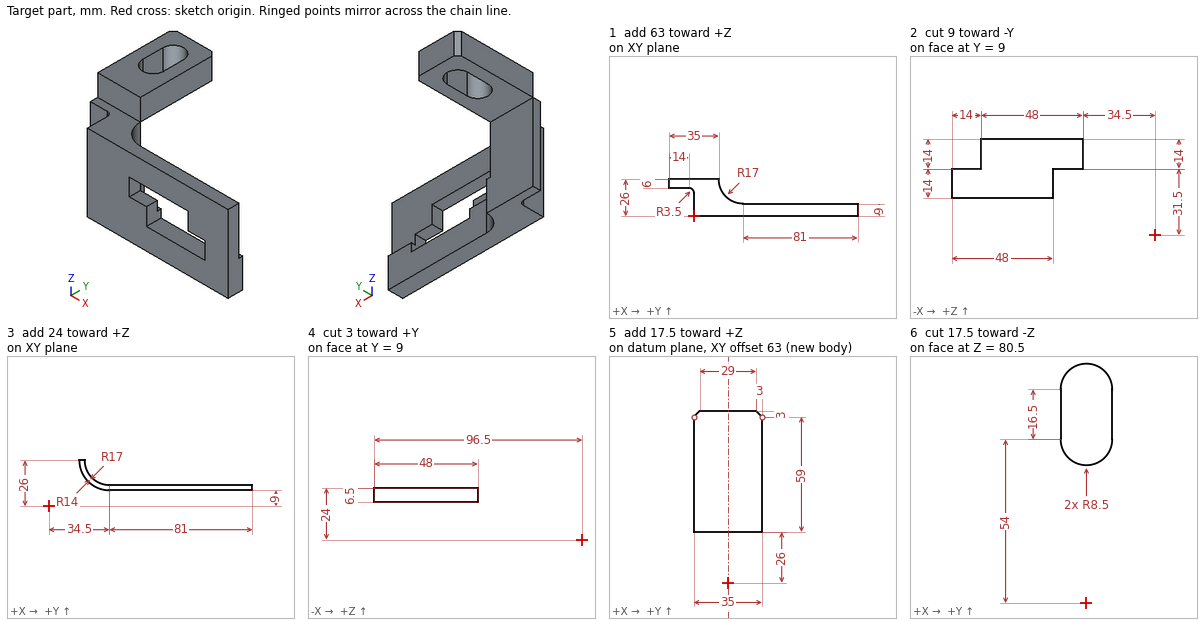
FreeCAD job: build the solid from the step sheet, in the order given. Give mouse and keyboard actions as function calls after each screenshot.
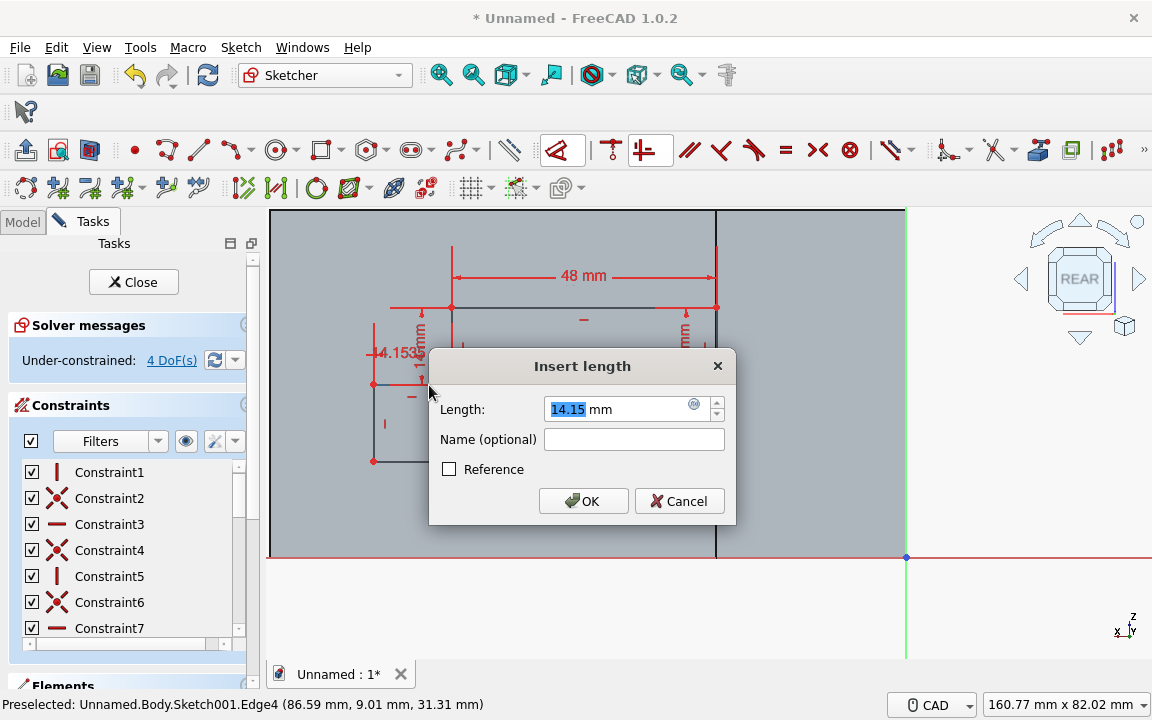
text(14)
key(Return)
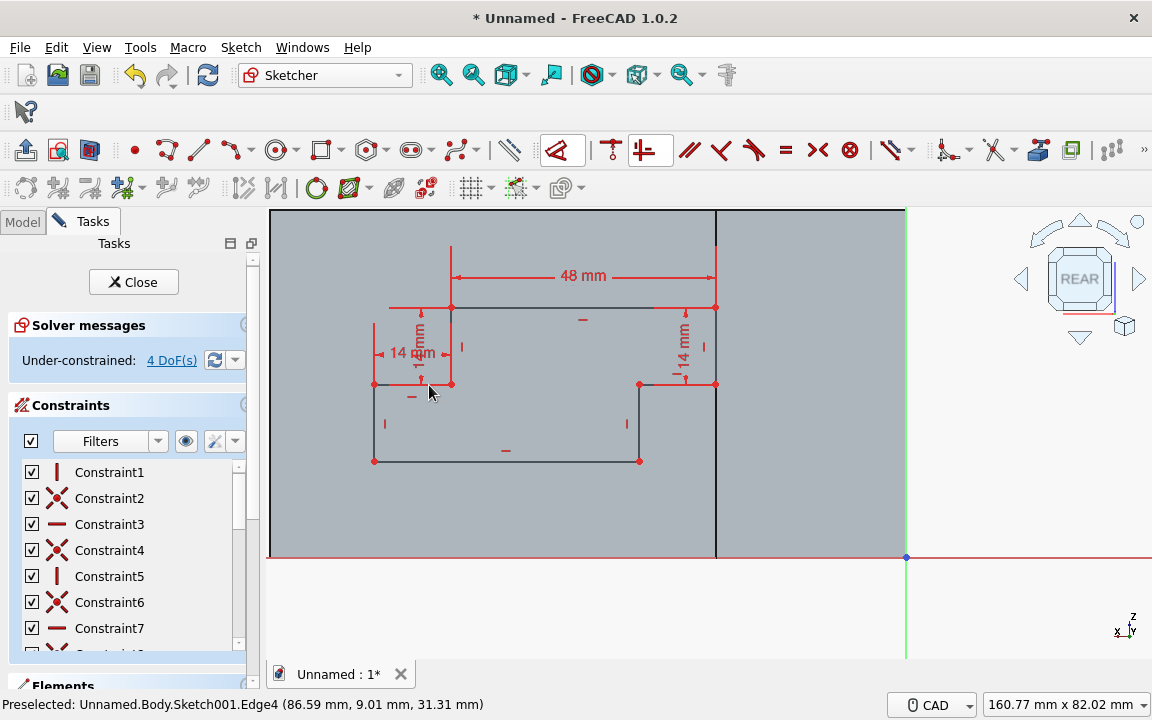
click(374, 408)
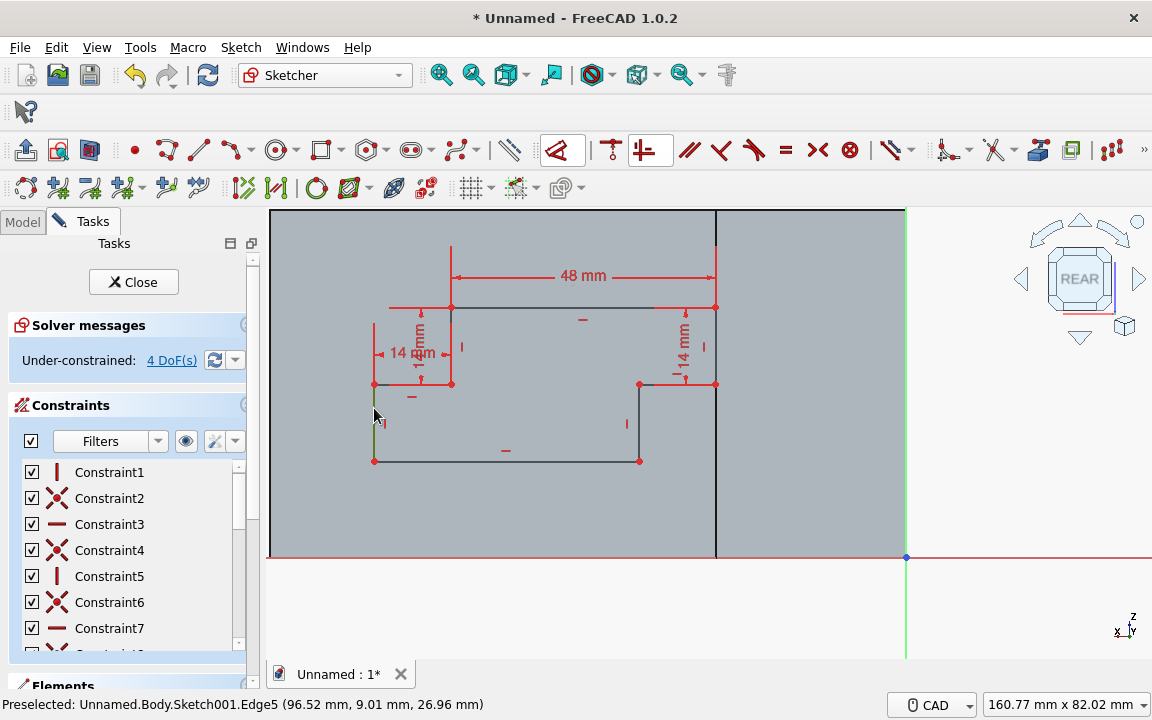
key(i)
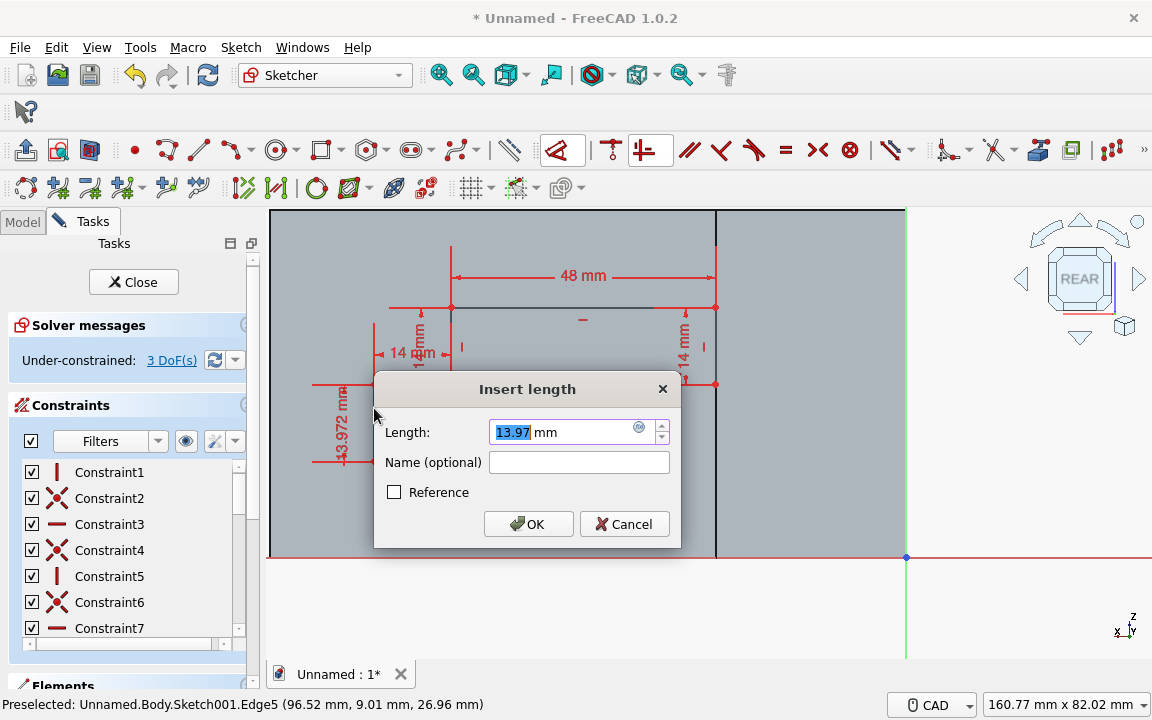
text(14)
key(Return)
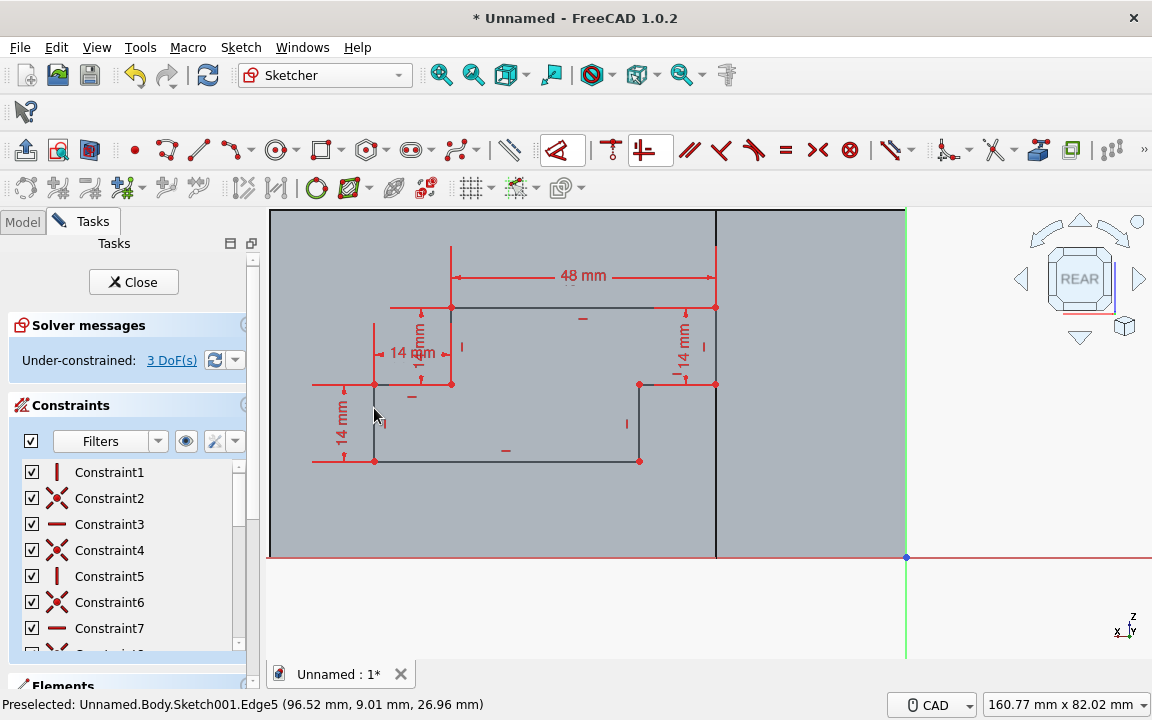
click(454, 462)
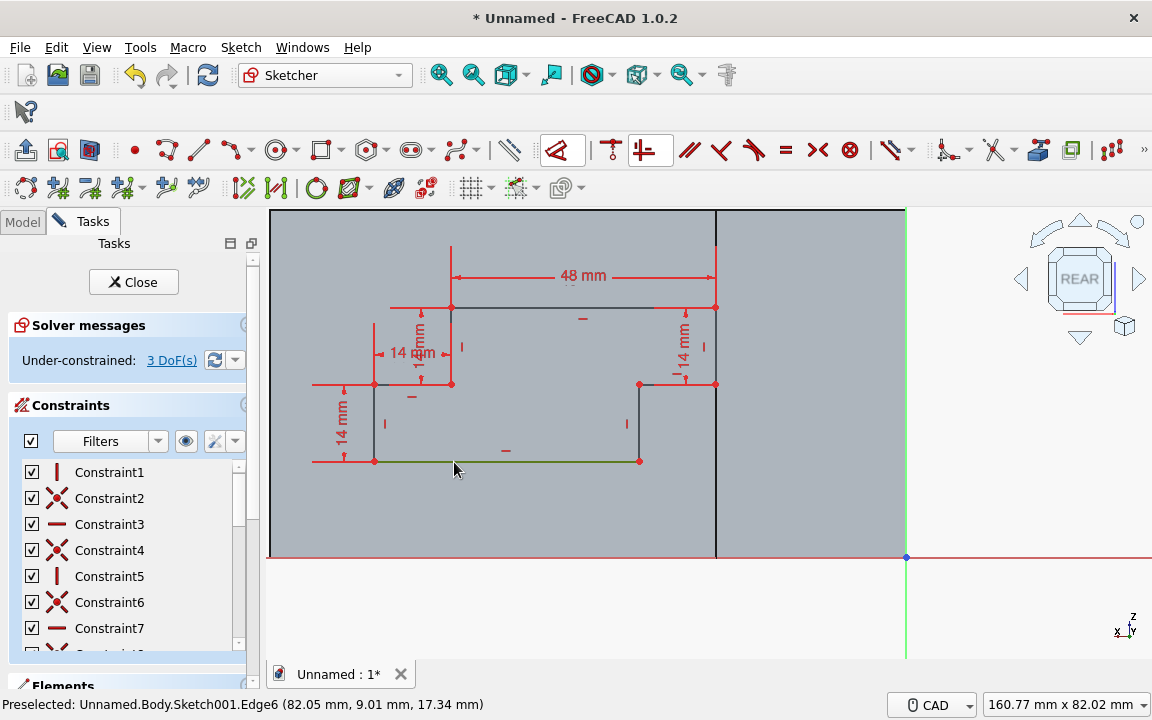
key(l)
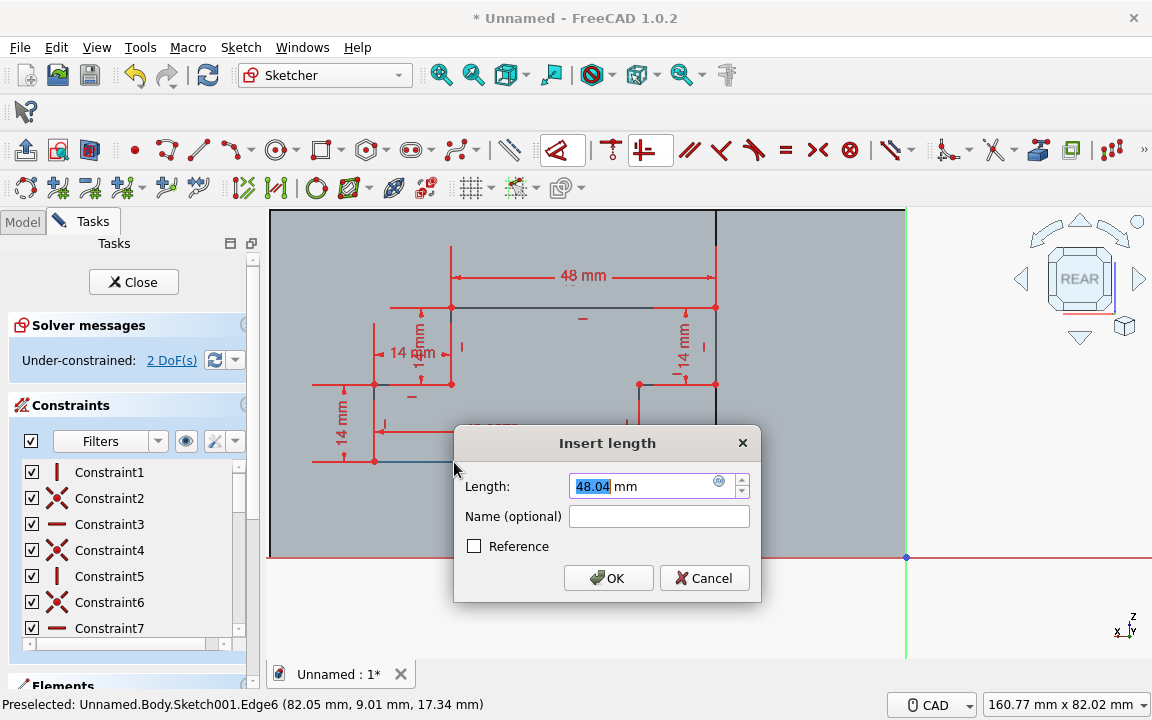
text(48)
key(Return)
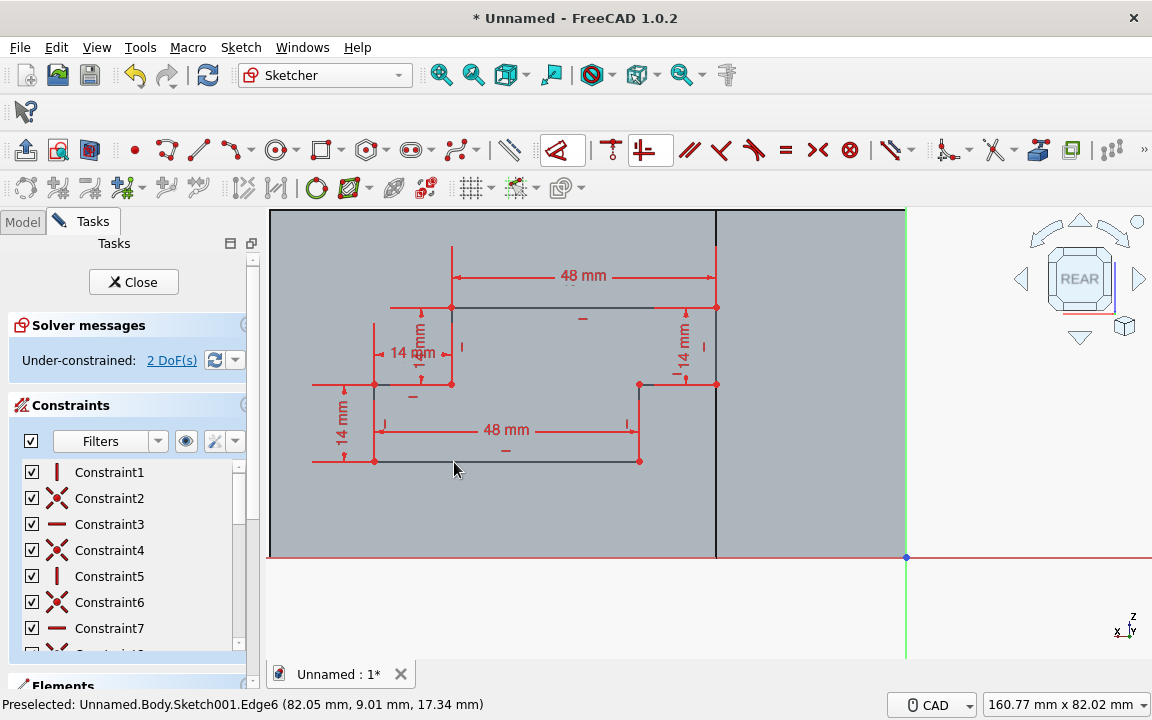
click(716, 385)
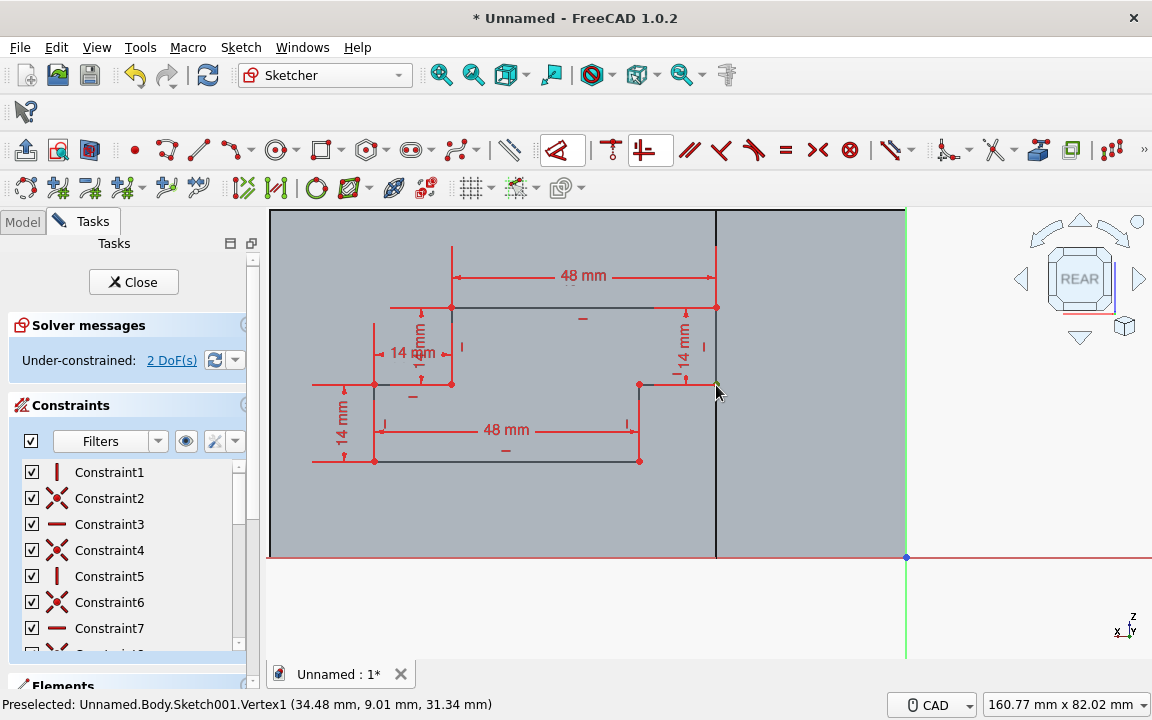
key(l)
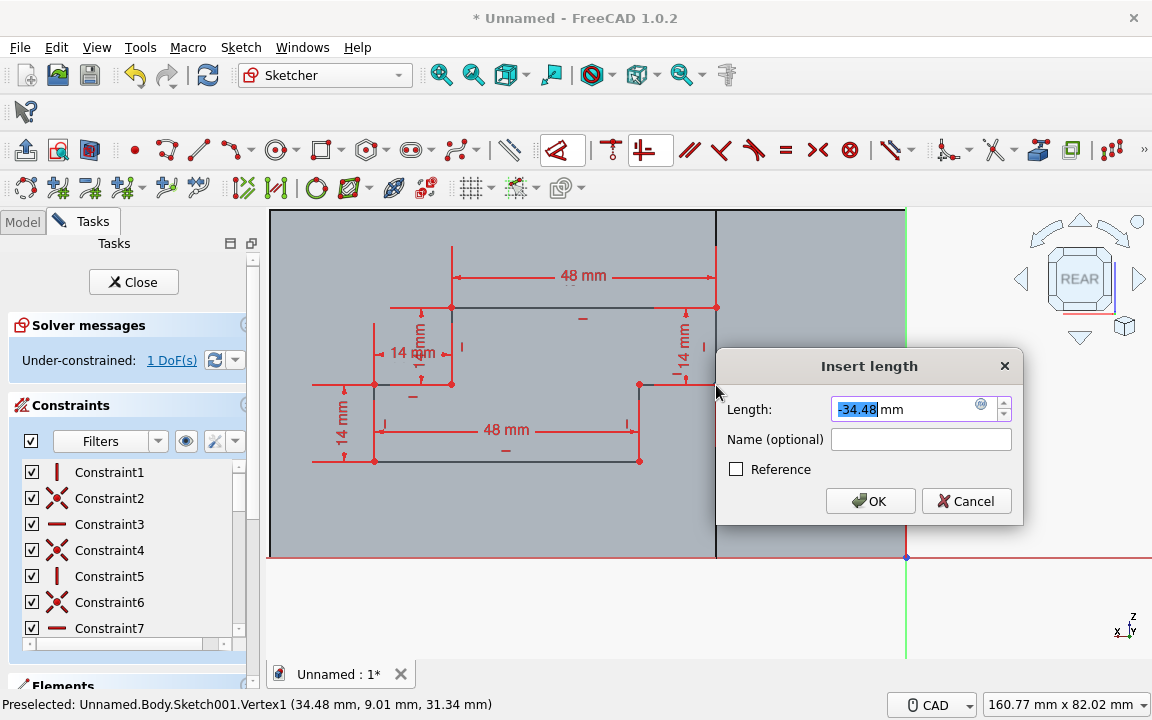
text(-34.5)
key(Return)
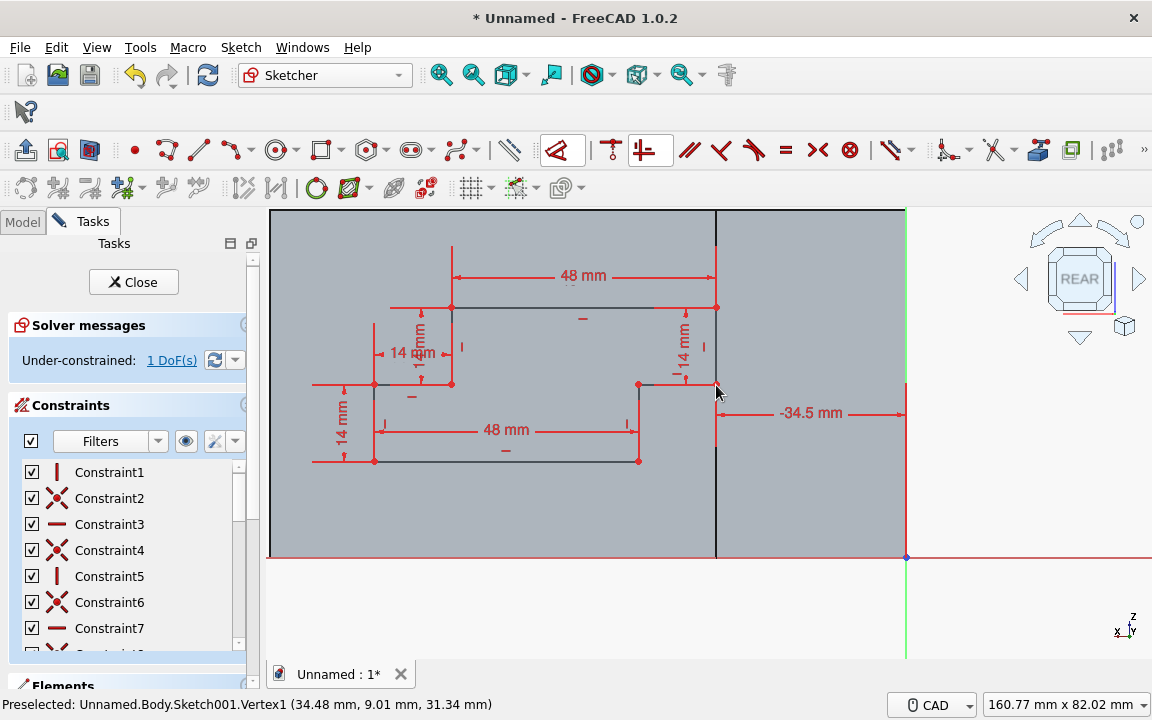
click(716, 385)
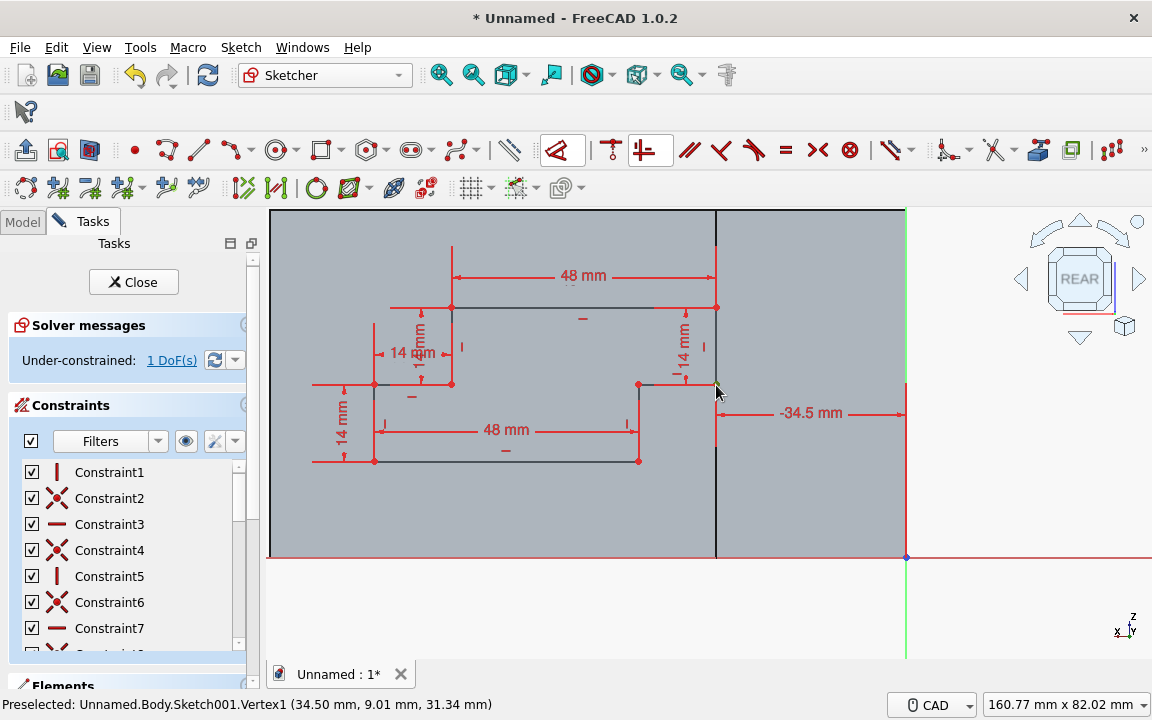
key(i)